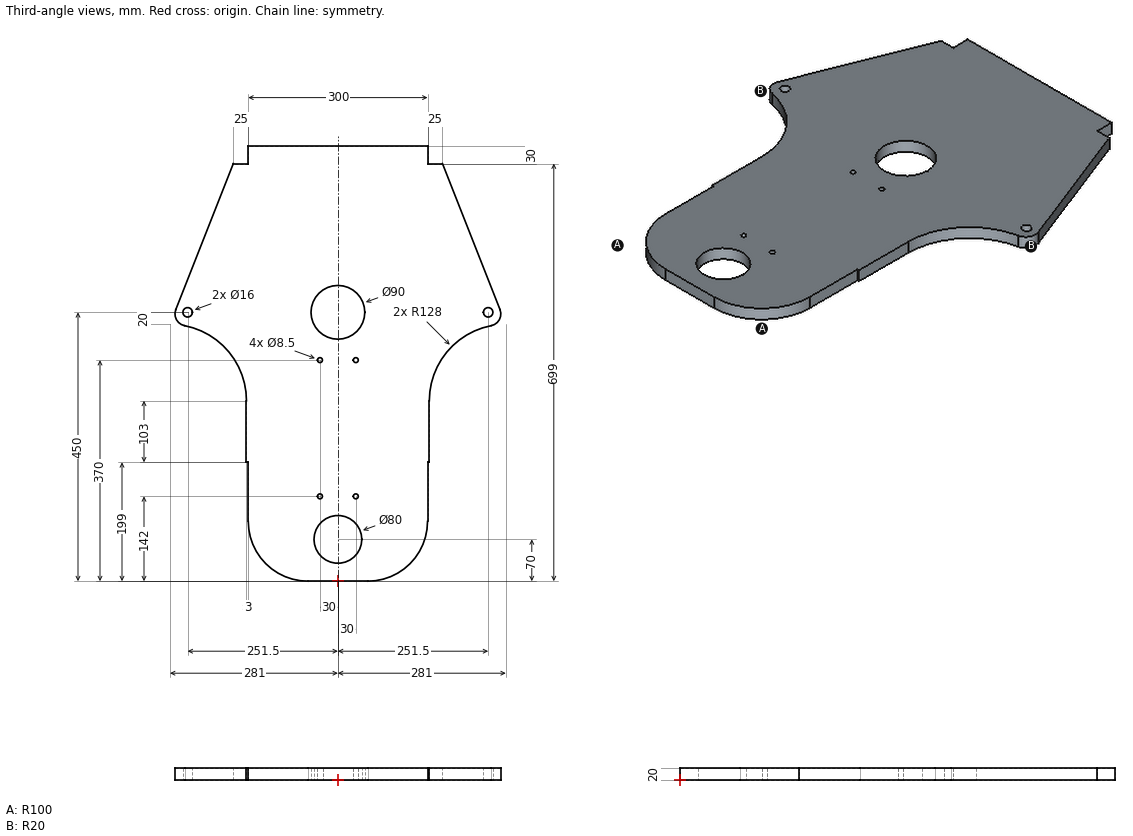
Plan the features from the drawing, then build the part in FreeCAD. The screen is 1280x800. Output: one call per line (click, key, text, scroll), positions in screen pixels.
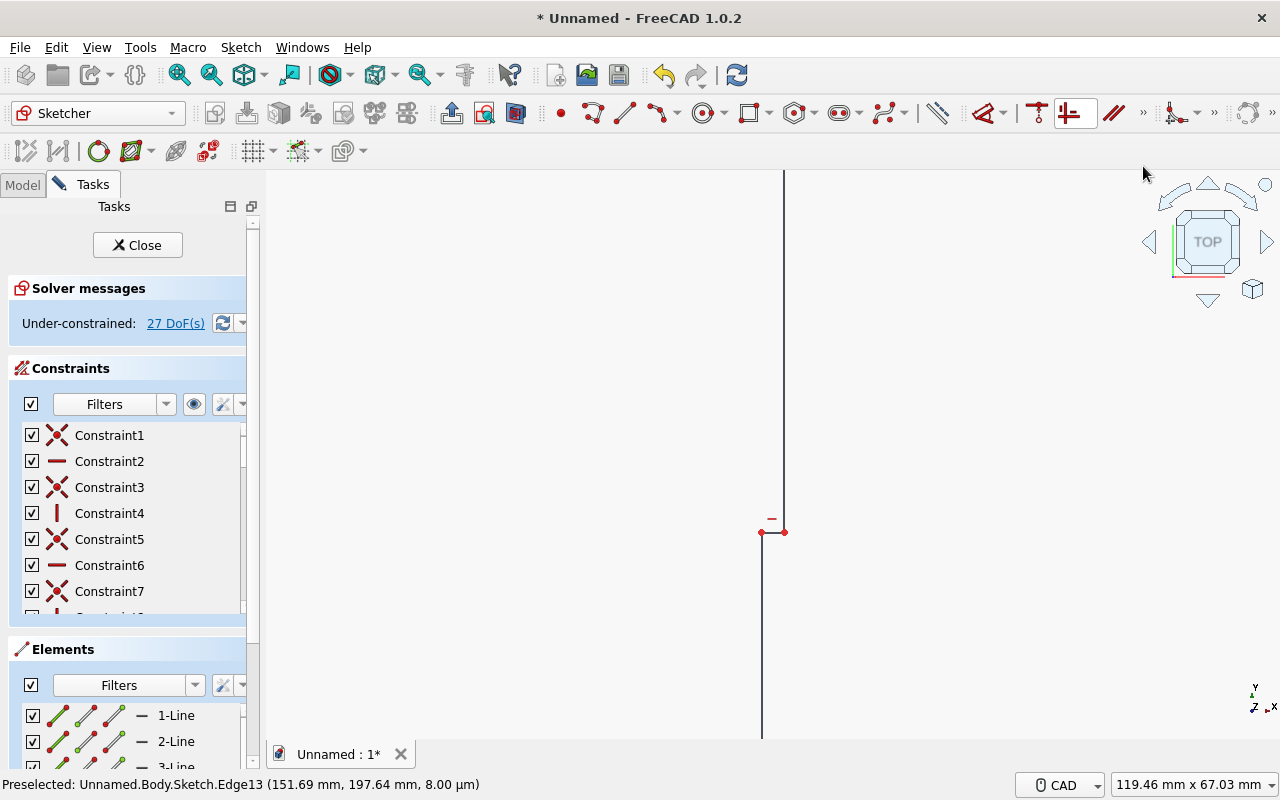
scroll(783, 542, down, 14)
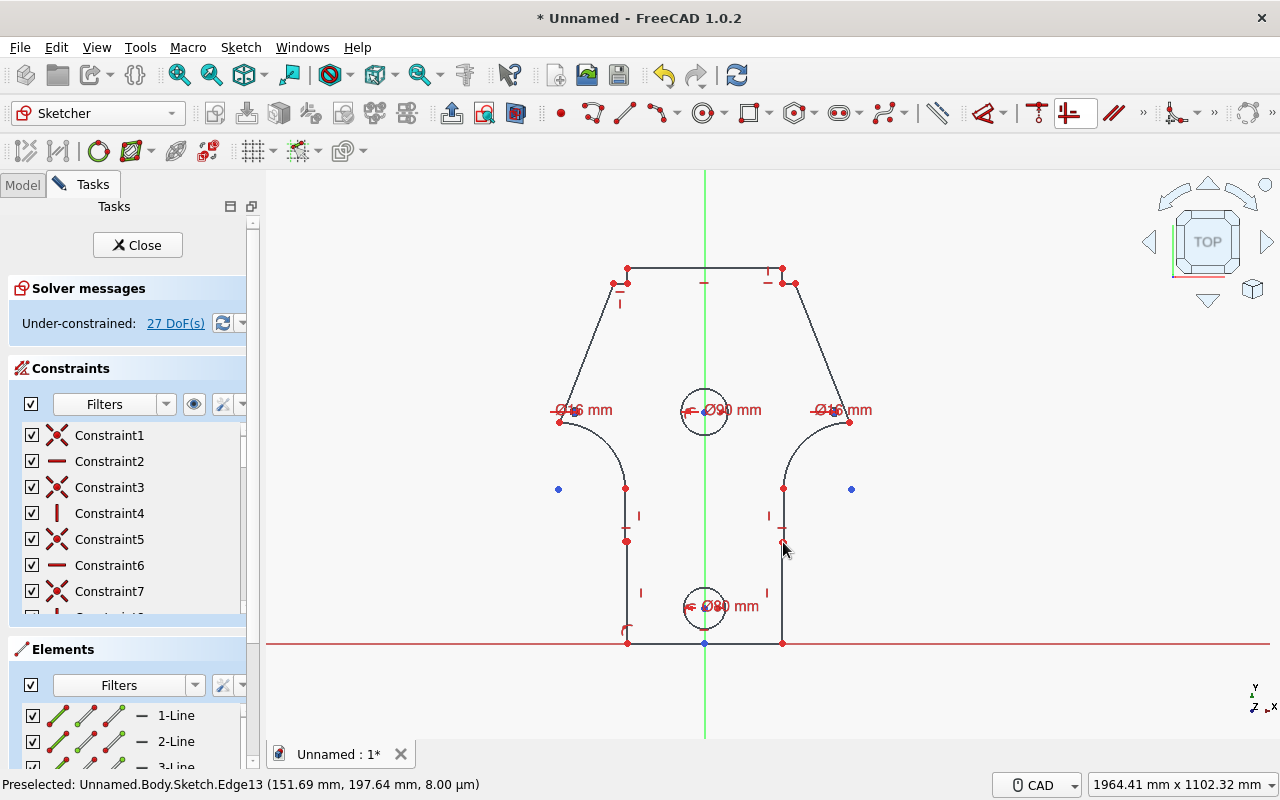
click(618, 459)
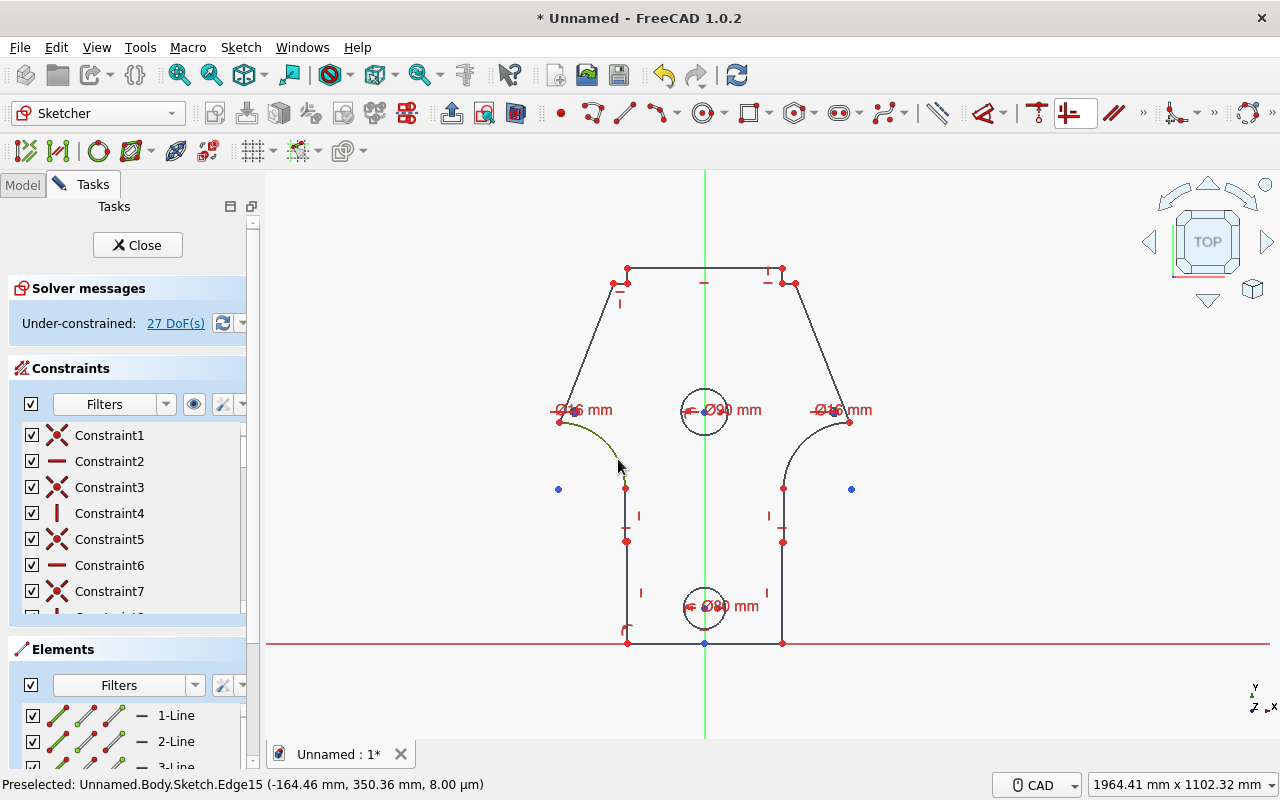
click(820, 430)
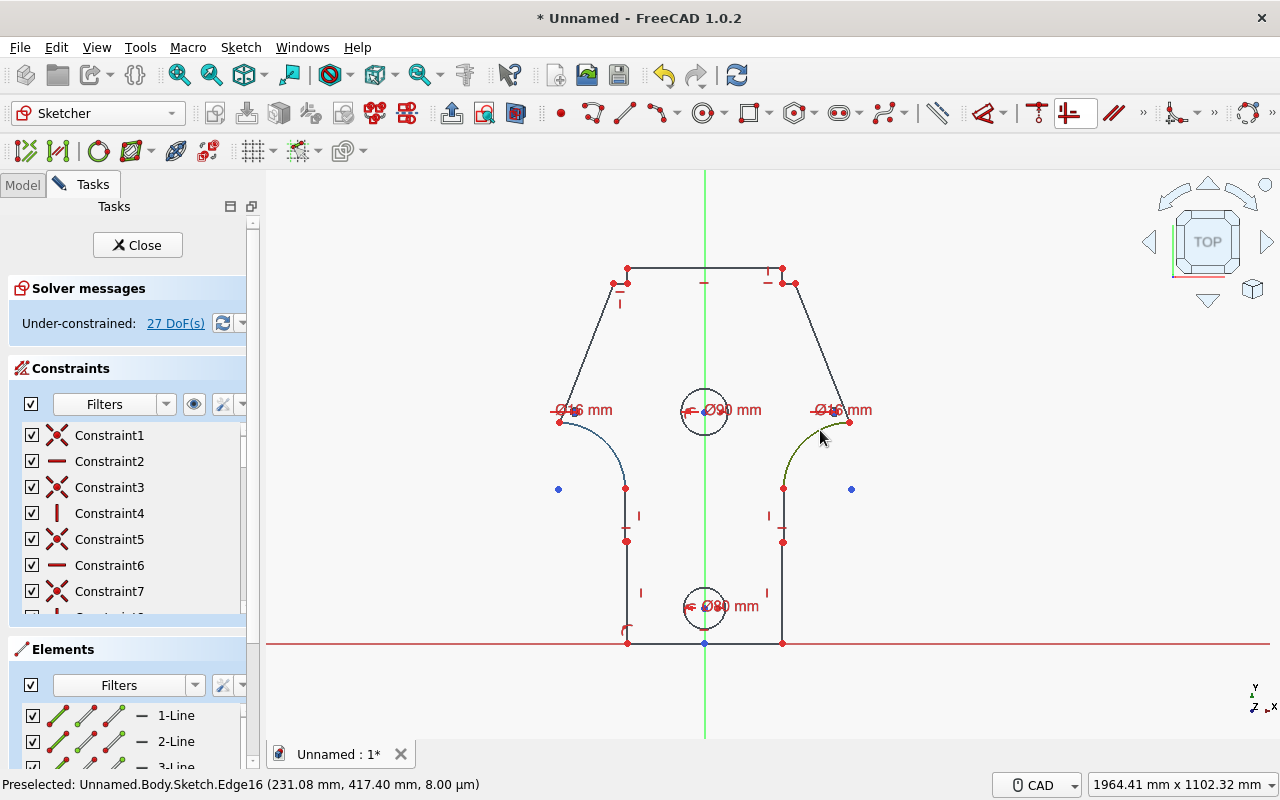
key(e)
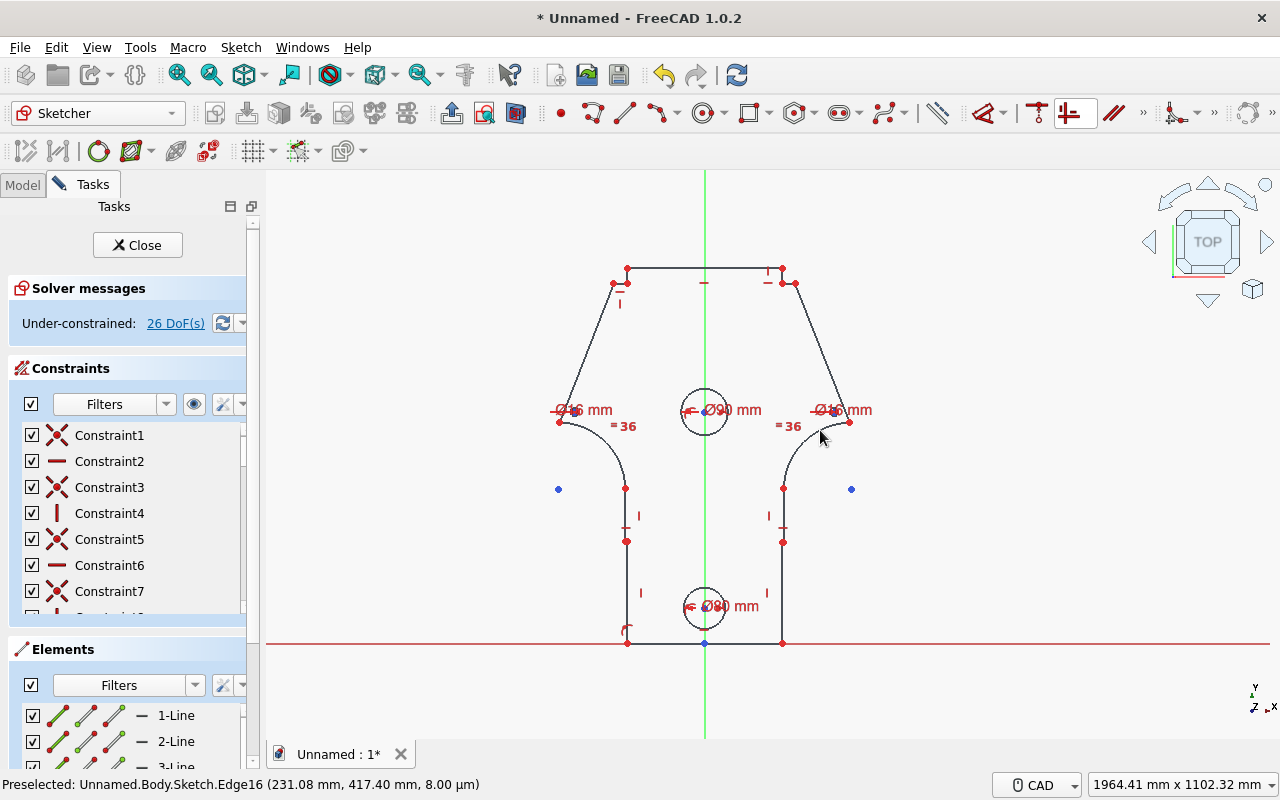
click(575, 412)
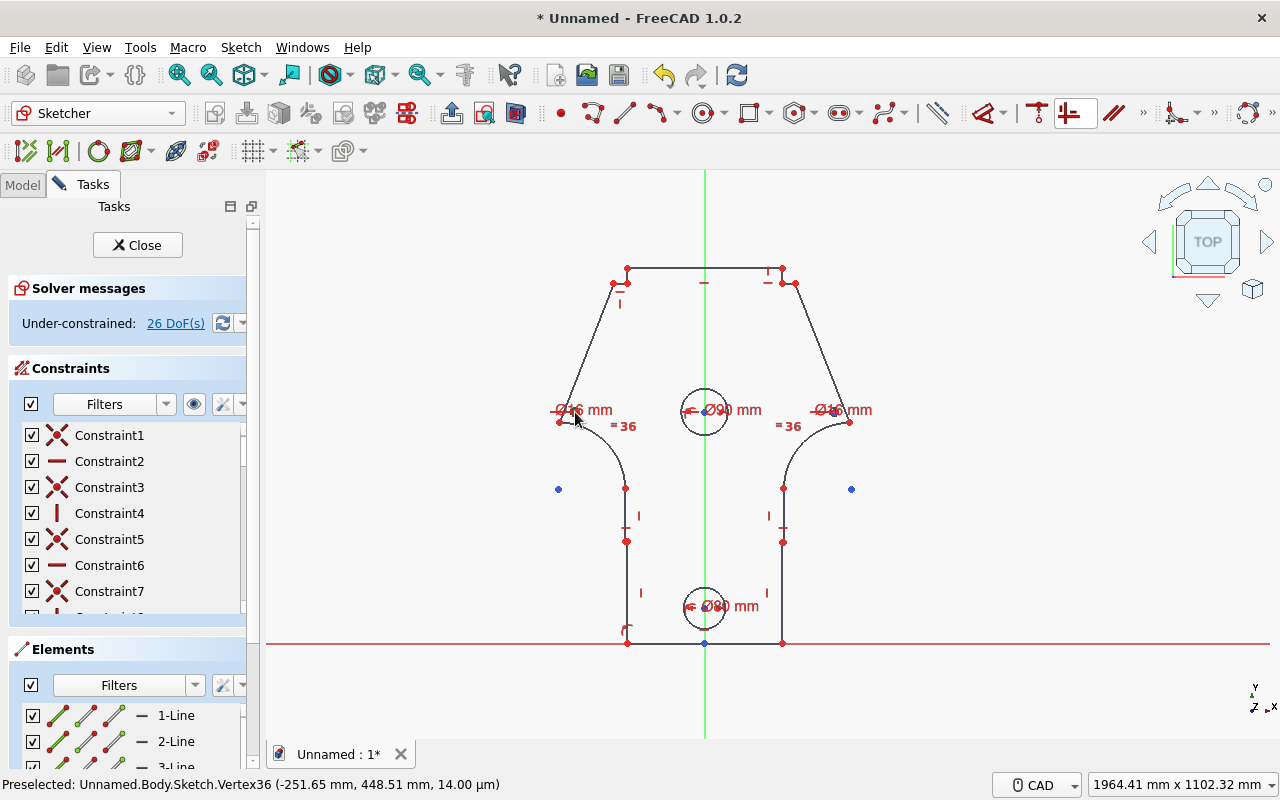
click(705, 412)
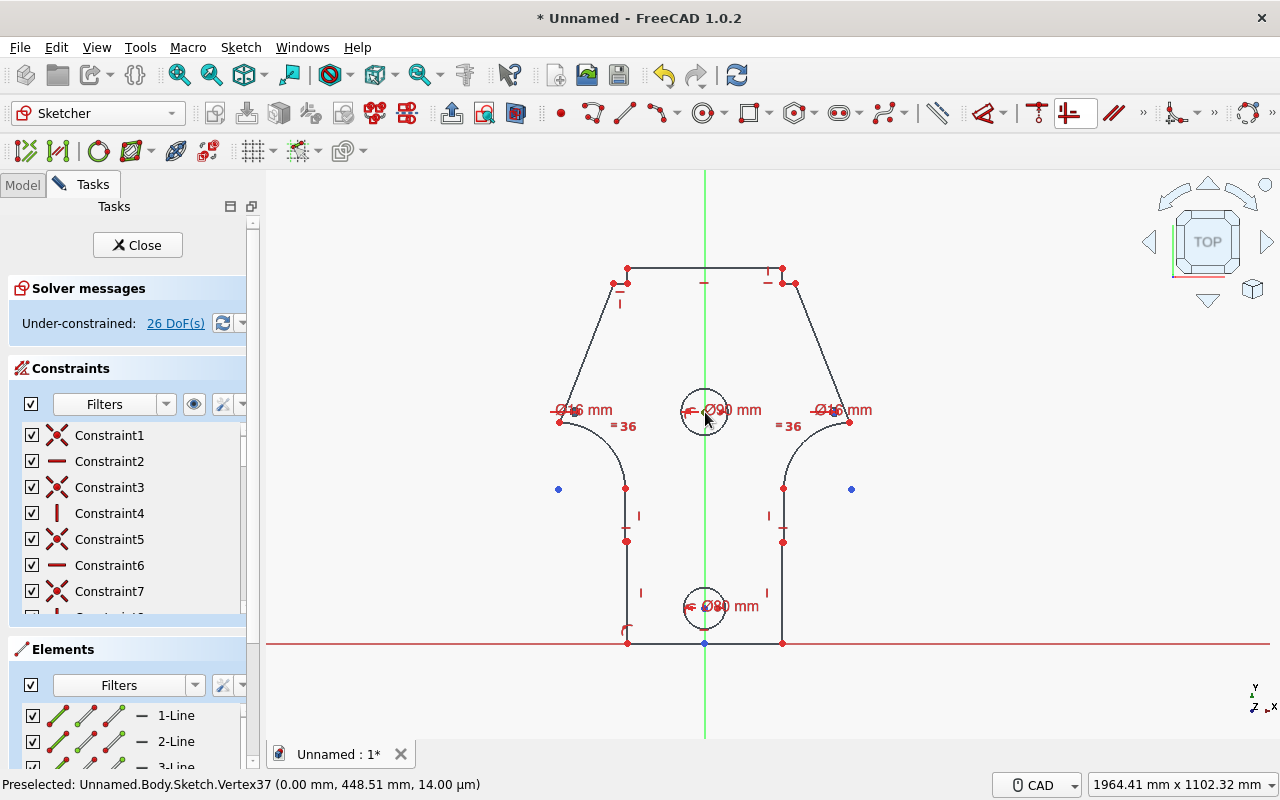
key(h)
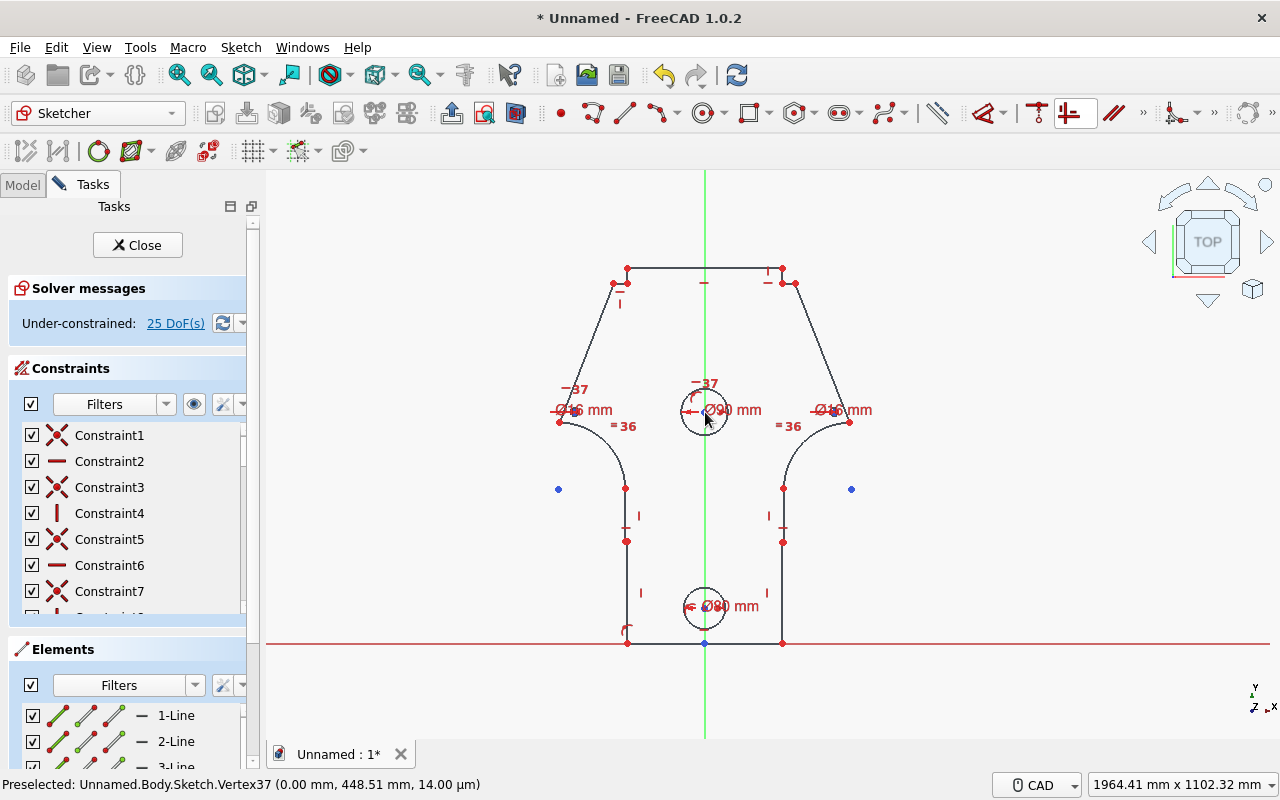
click(705, 412)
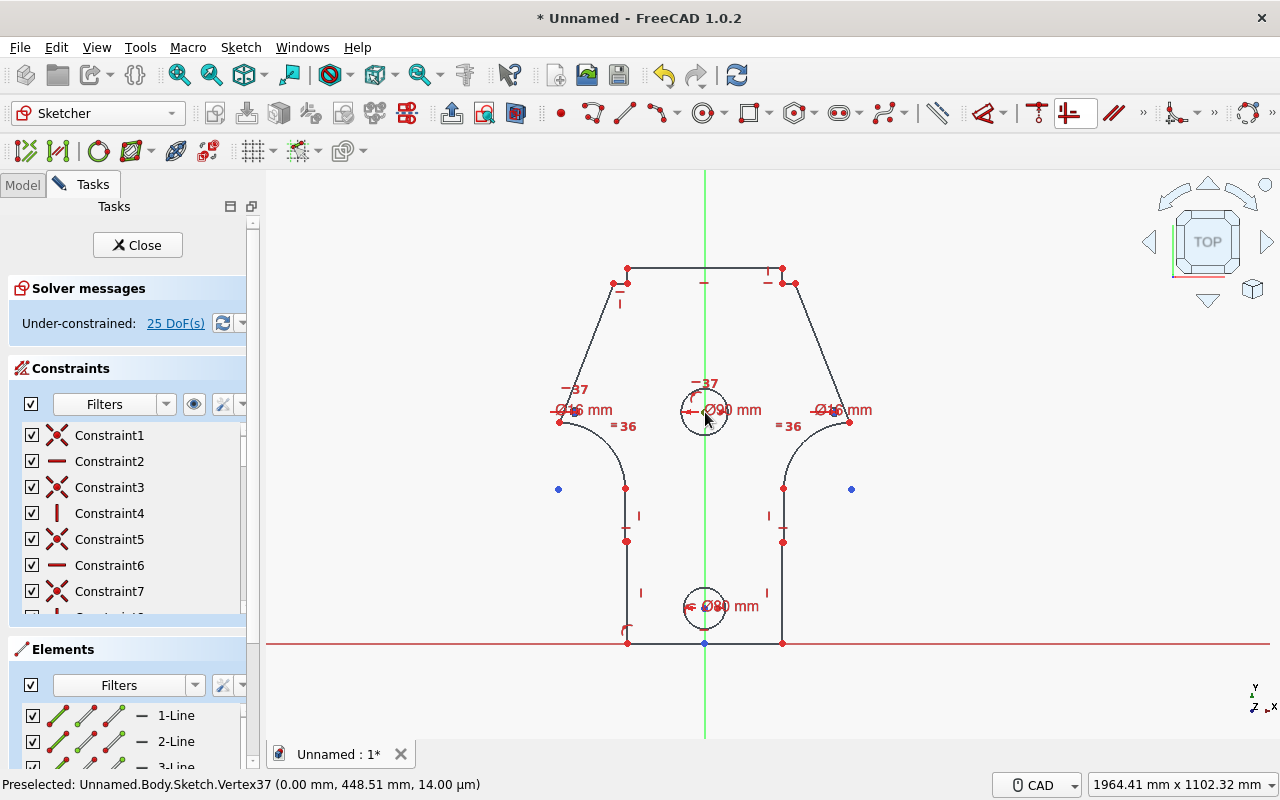
click(834, 412)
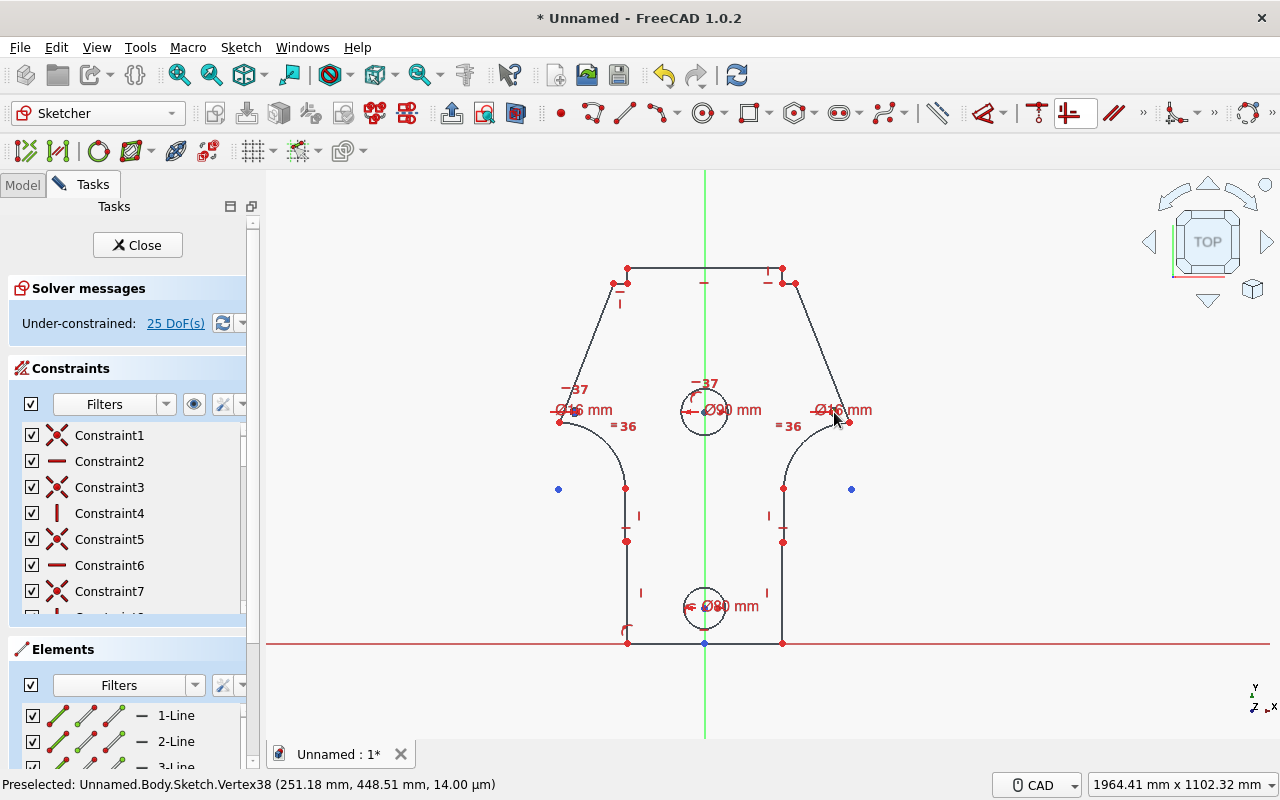
key(h)